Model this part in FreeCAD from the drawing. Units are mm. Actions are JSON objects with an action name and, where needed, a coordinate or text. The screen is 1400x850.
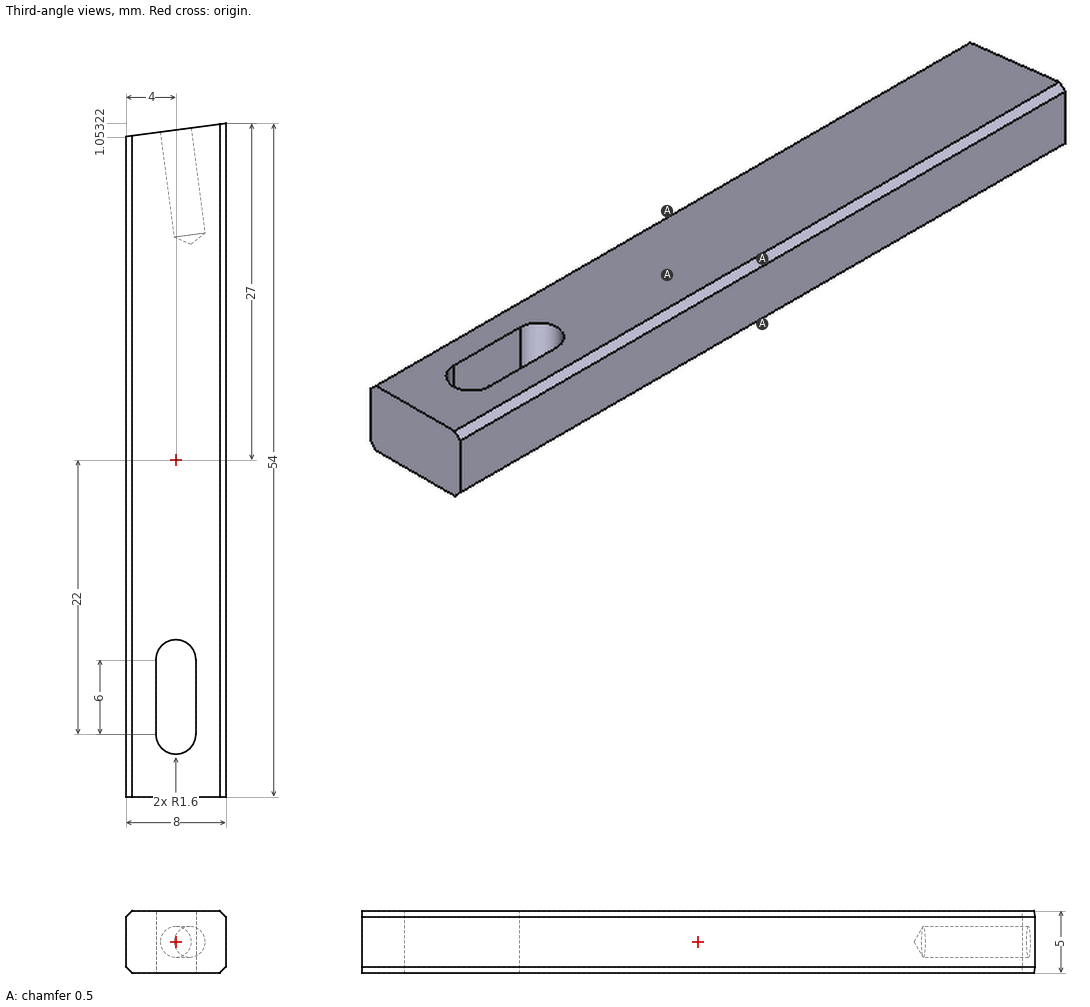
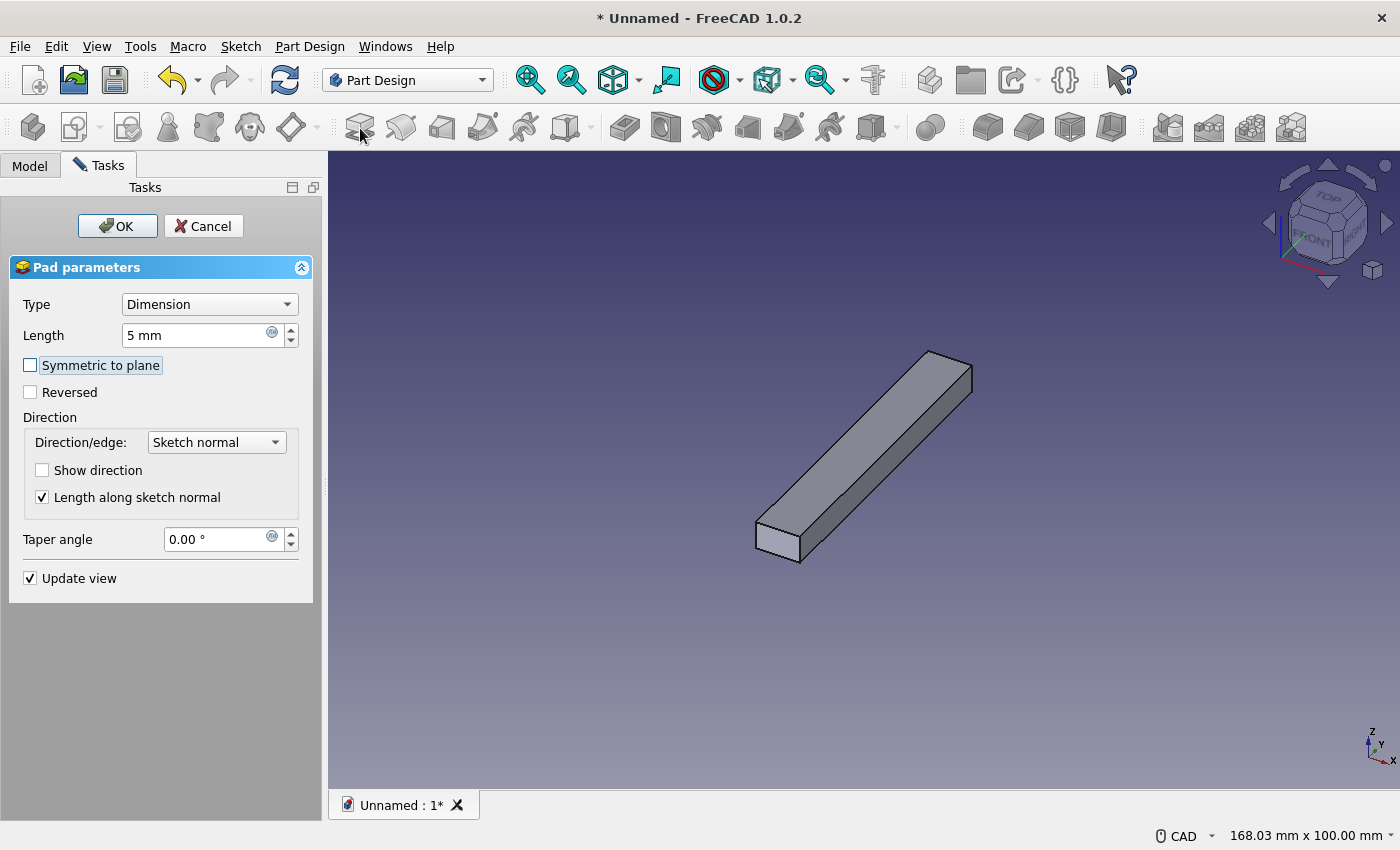
{"action": "left_click", "coordinate": [31, 365]}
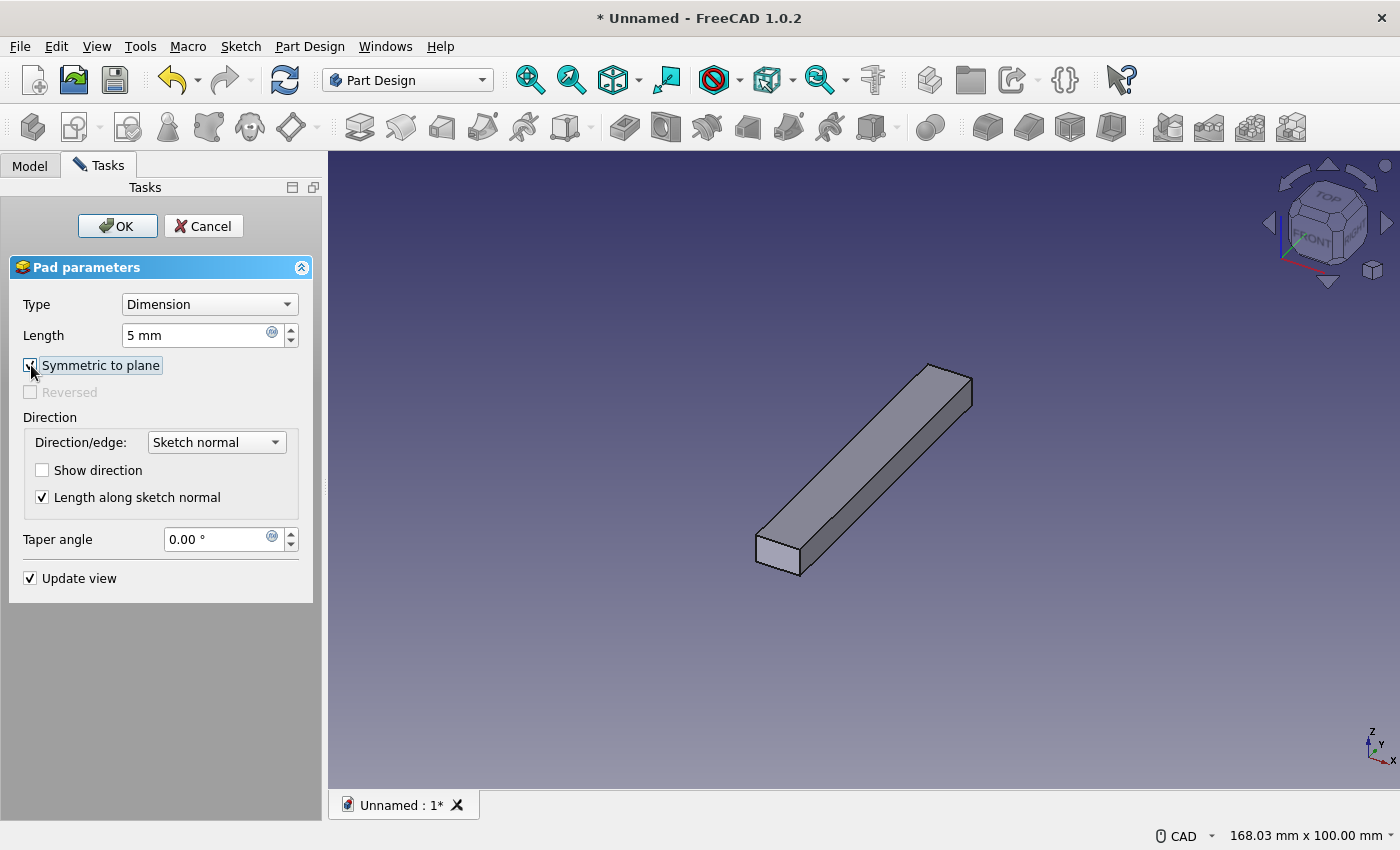
{"action": "left_click", "coordinate": [118, 226]}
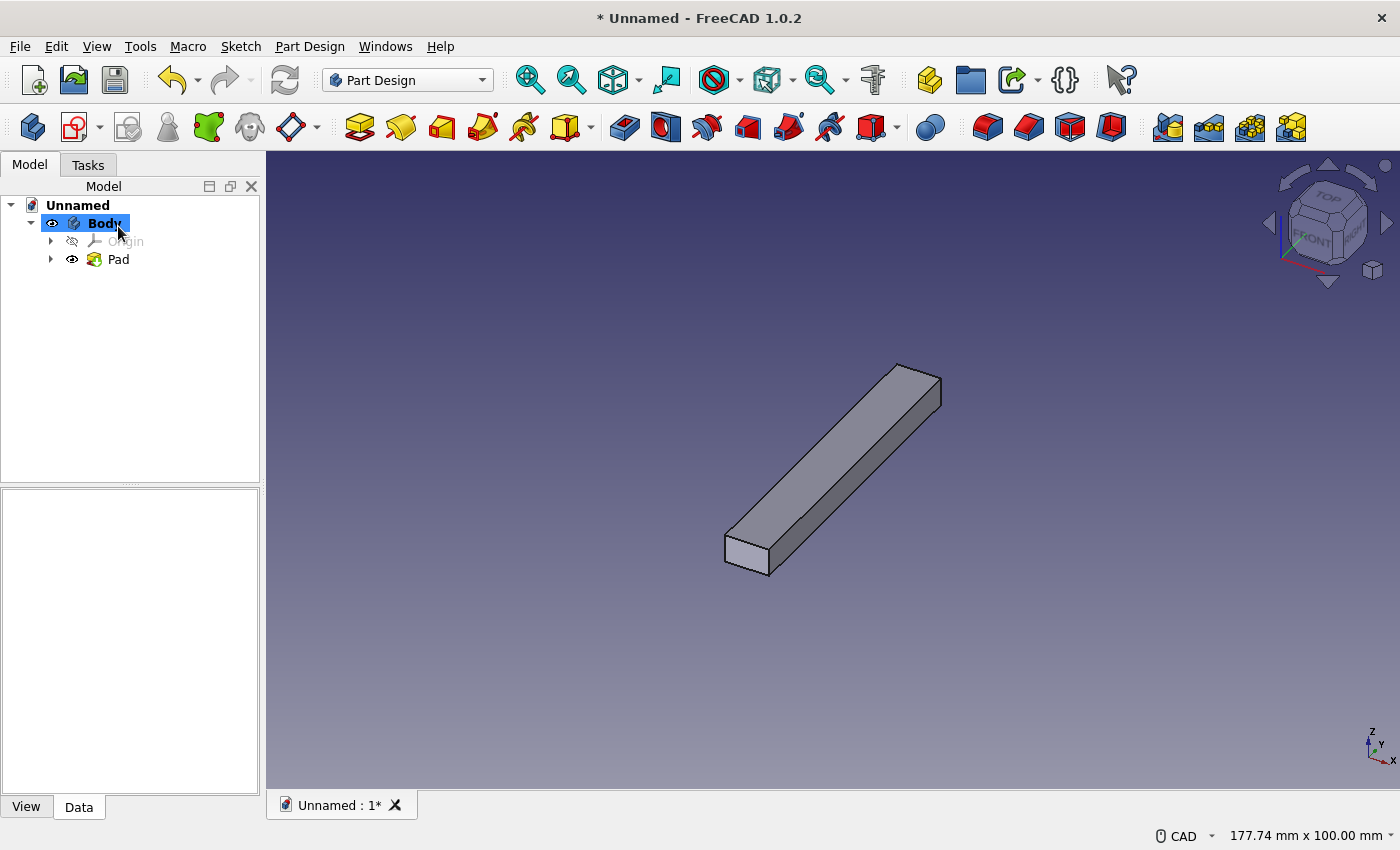
{"action": "left_click", "coordinate": [531, 80]}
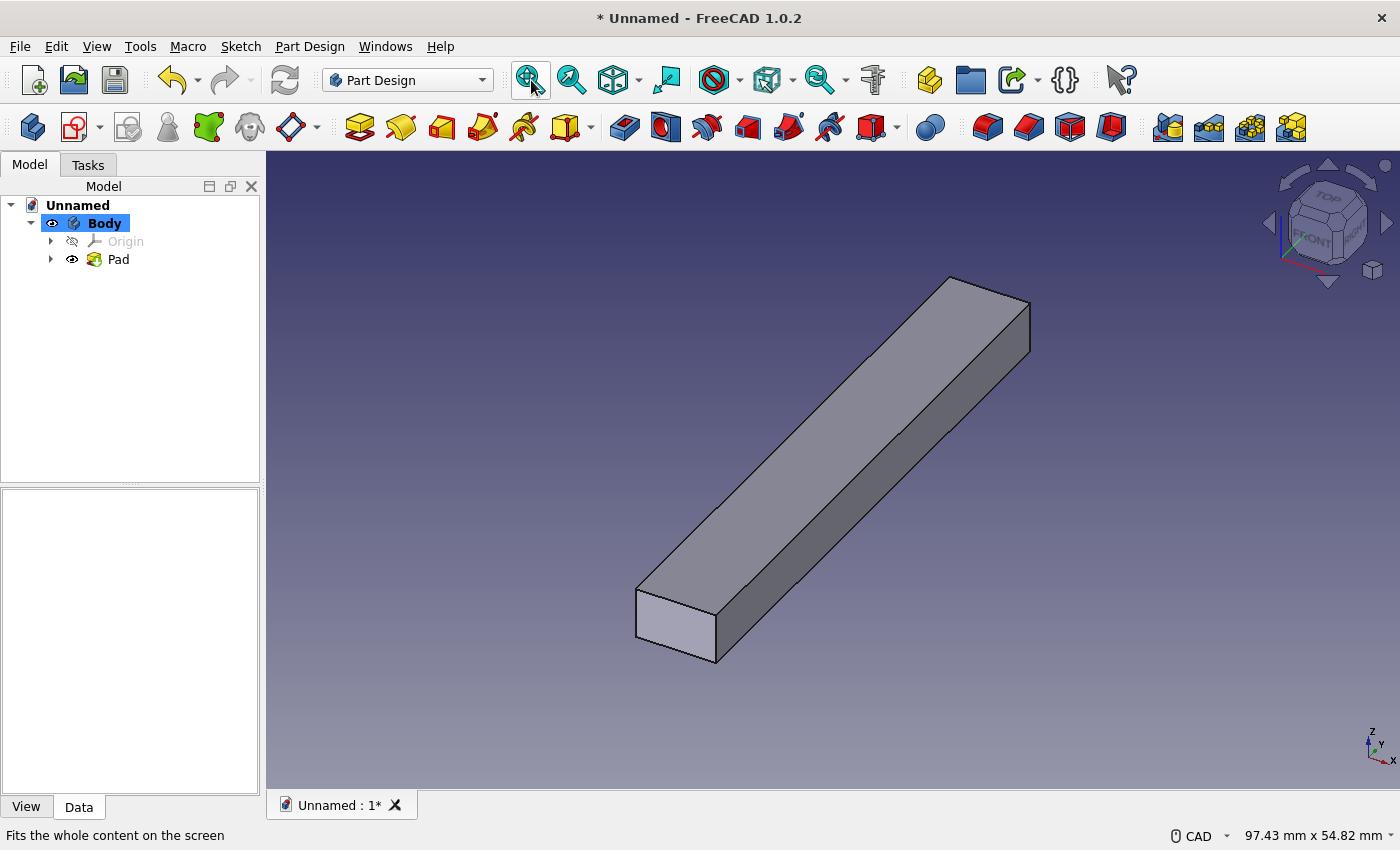
{"action": "left_click", "coordinate": [923, 356]}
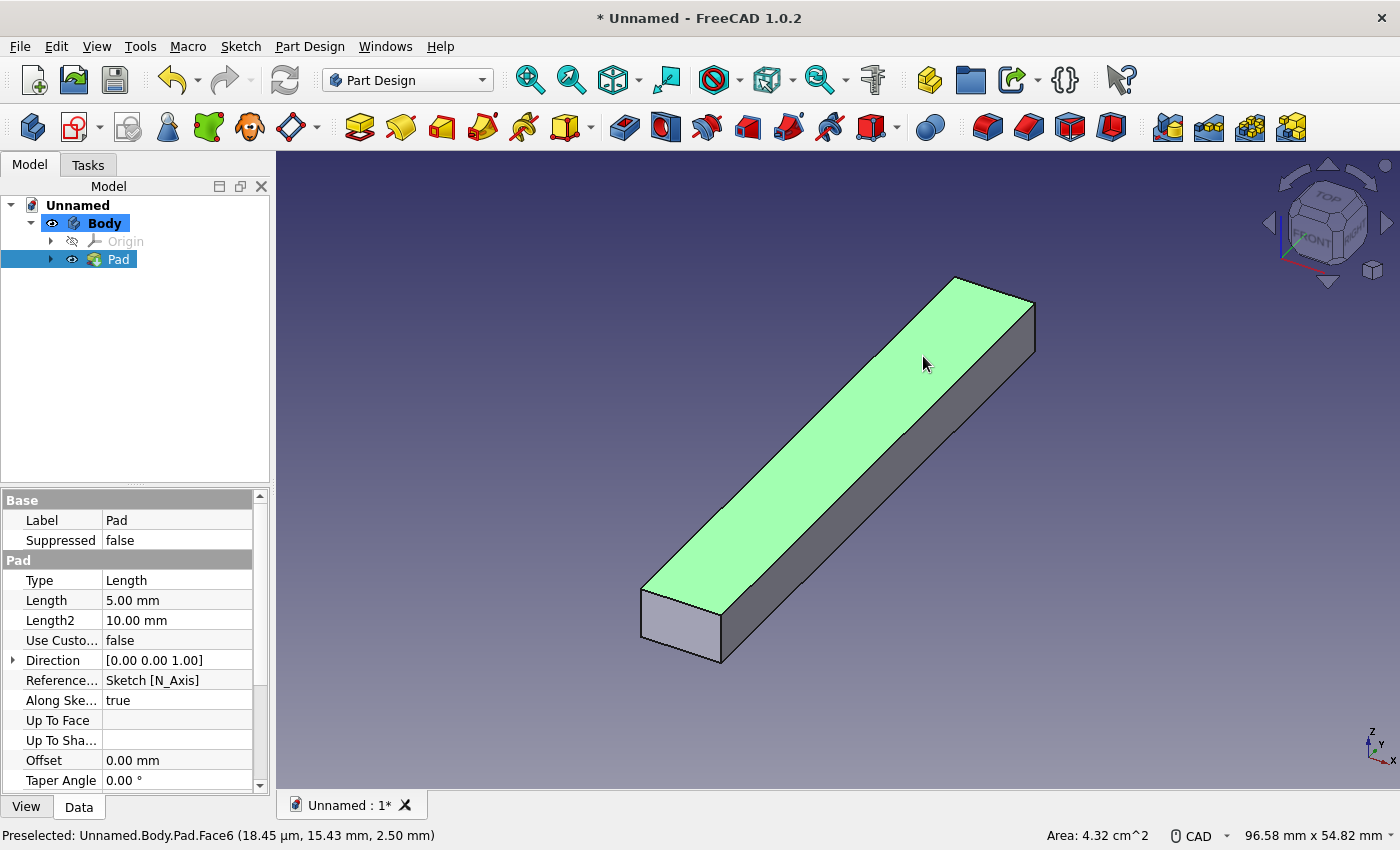
{"action": "left_click", "coordinate": [74, 128]}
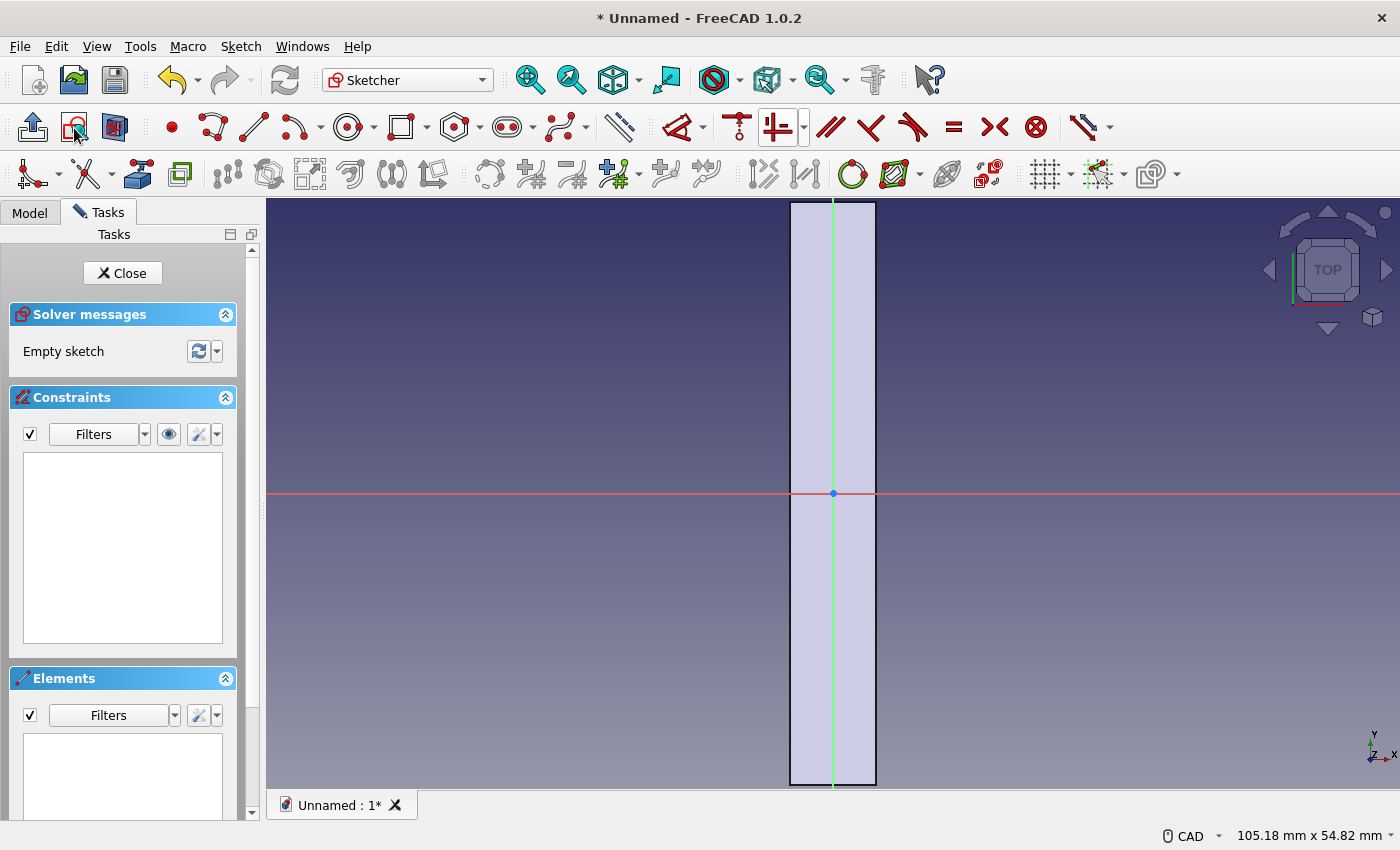
{"action": "scroll", "coordinate": [764, 494], "scroll_direction": "down", "scroll_amount": 5}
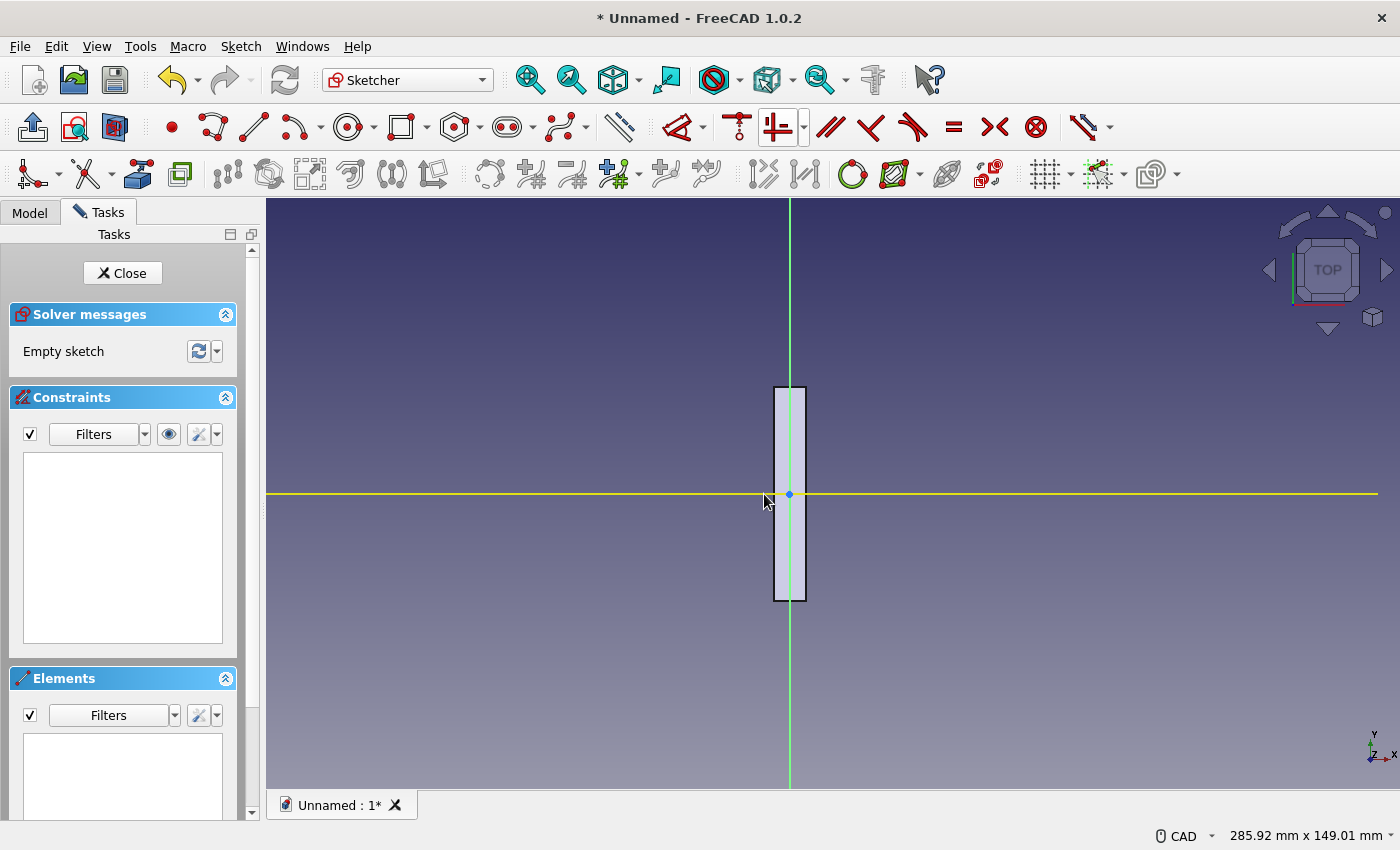
{"action": "scroll", "coordinate": [791, 384], "scroll_direction": "up", "scroll_amount": 15}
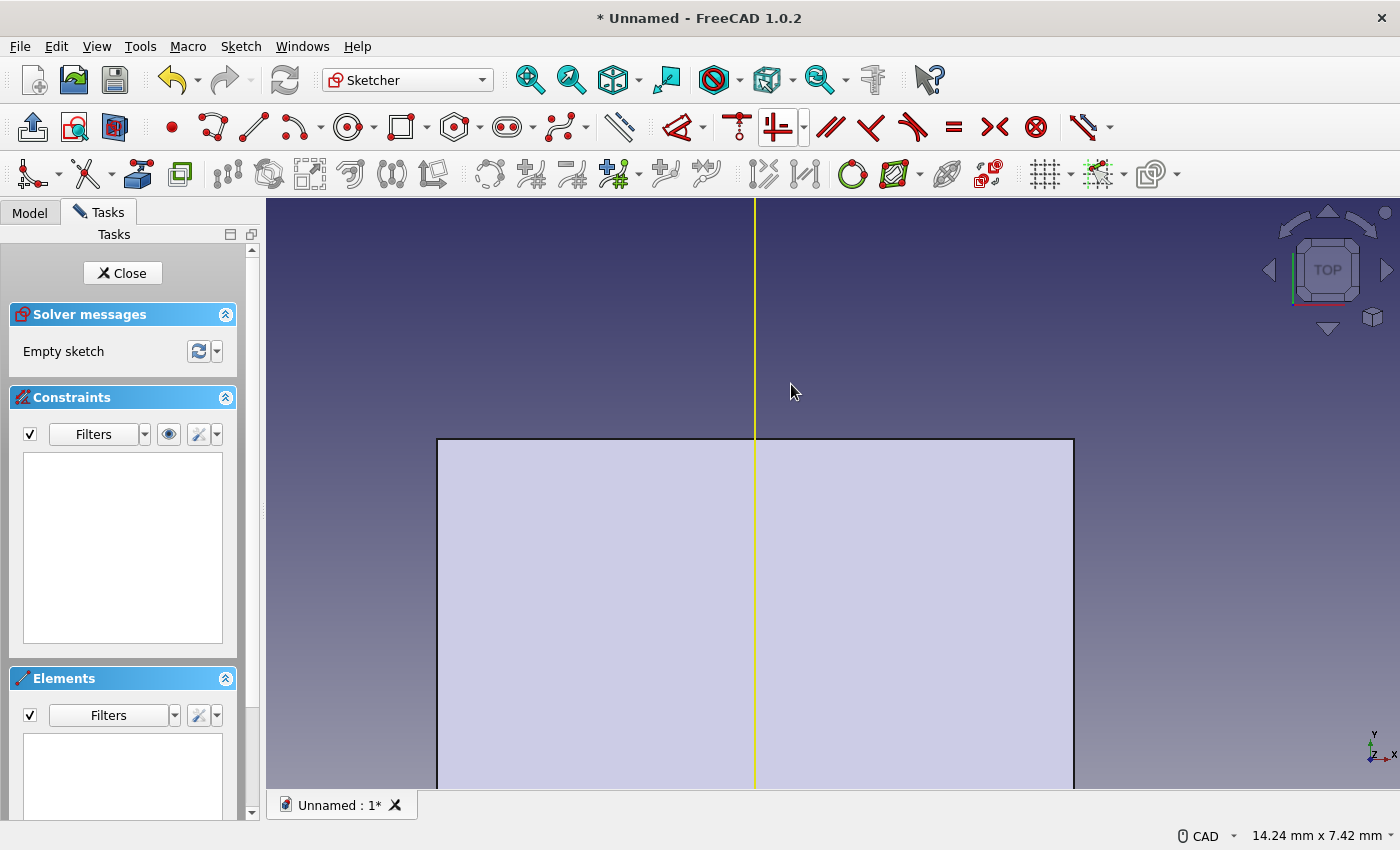
{"action": "key", "text": "g m"}